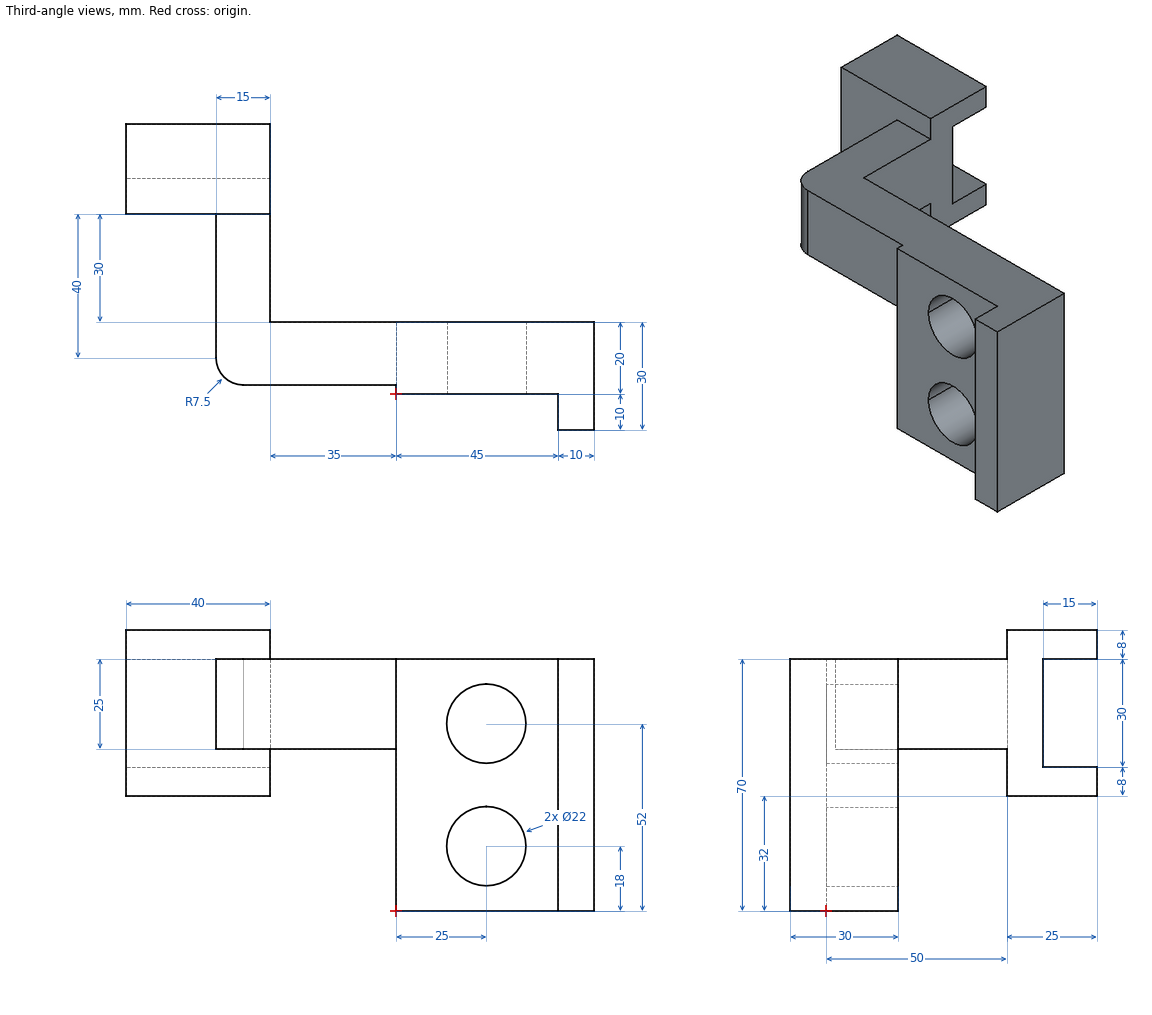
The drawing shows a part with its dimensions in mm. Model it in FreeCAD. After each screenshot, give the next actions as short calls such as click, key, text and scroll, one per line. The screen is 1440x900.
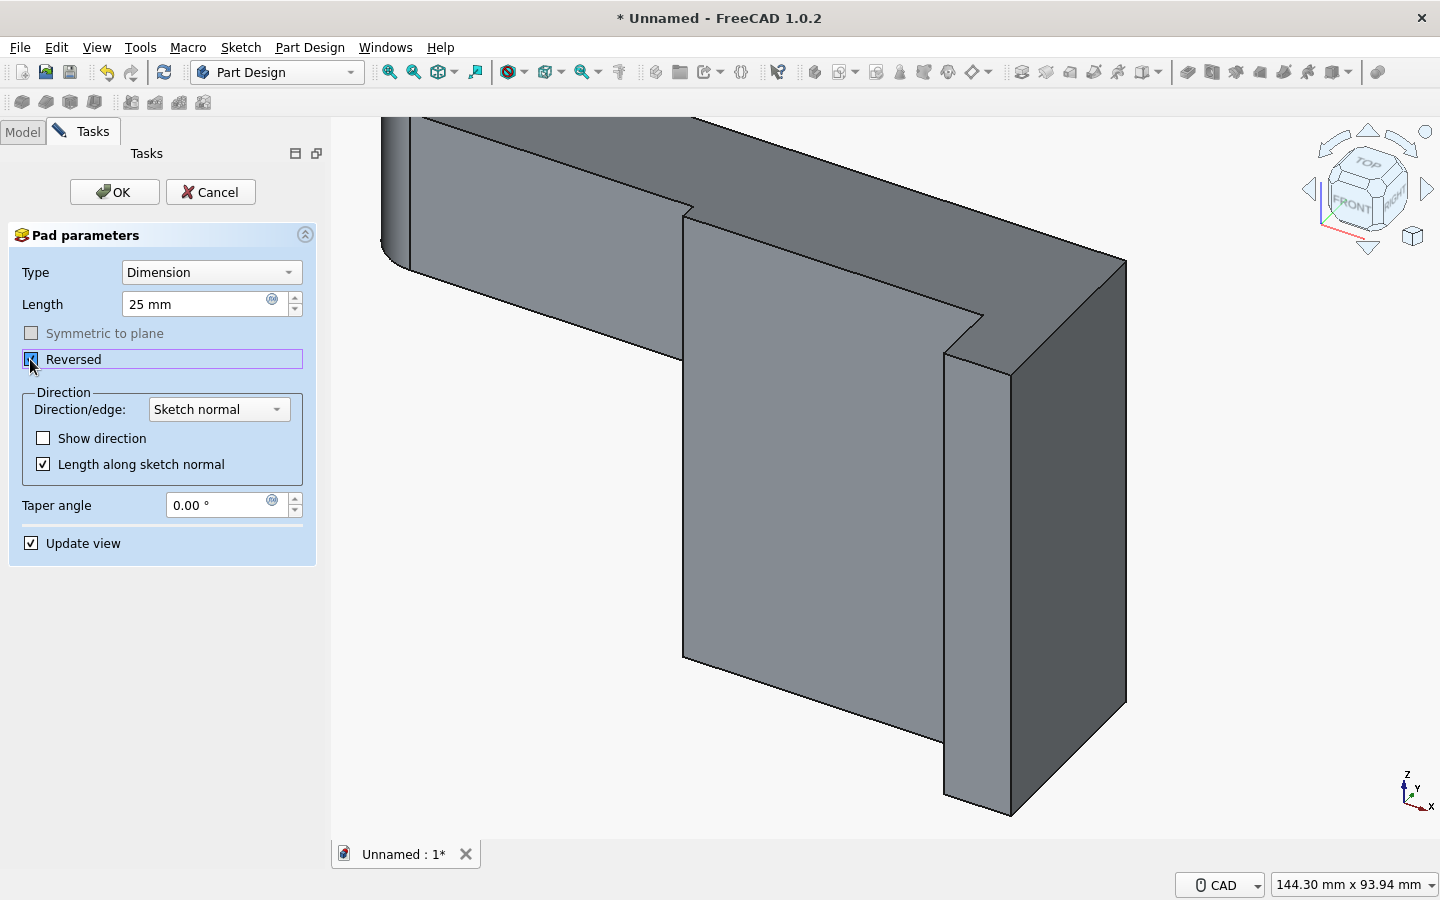
click(115, 192)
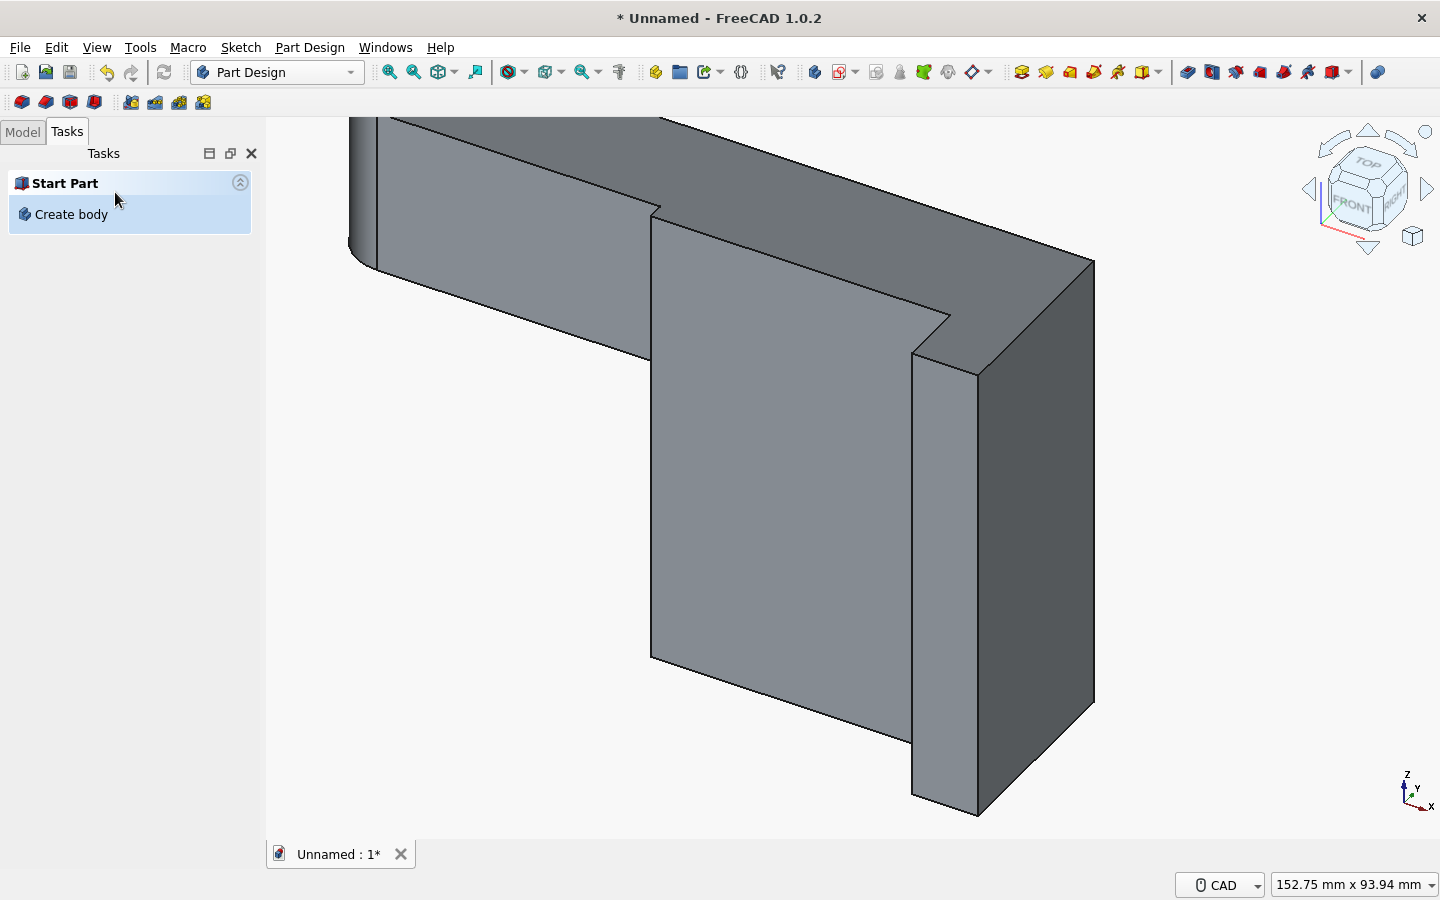
click(390, 72)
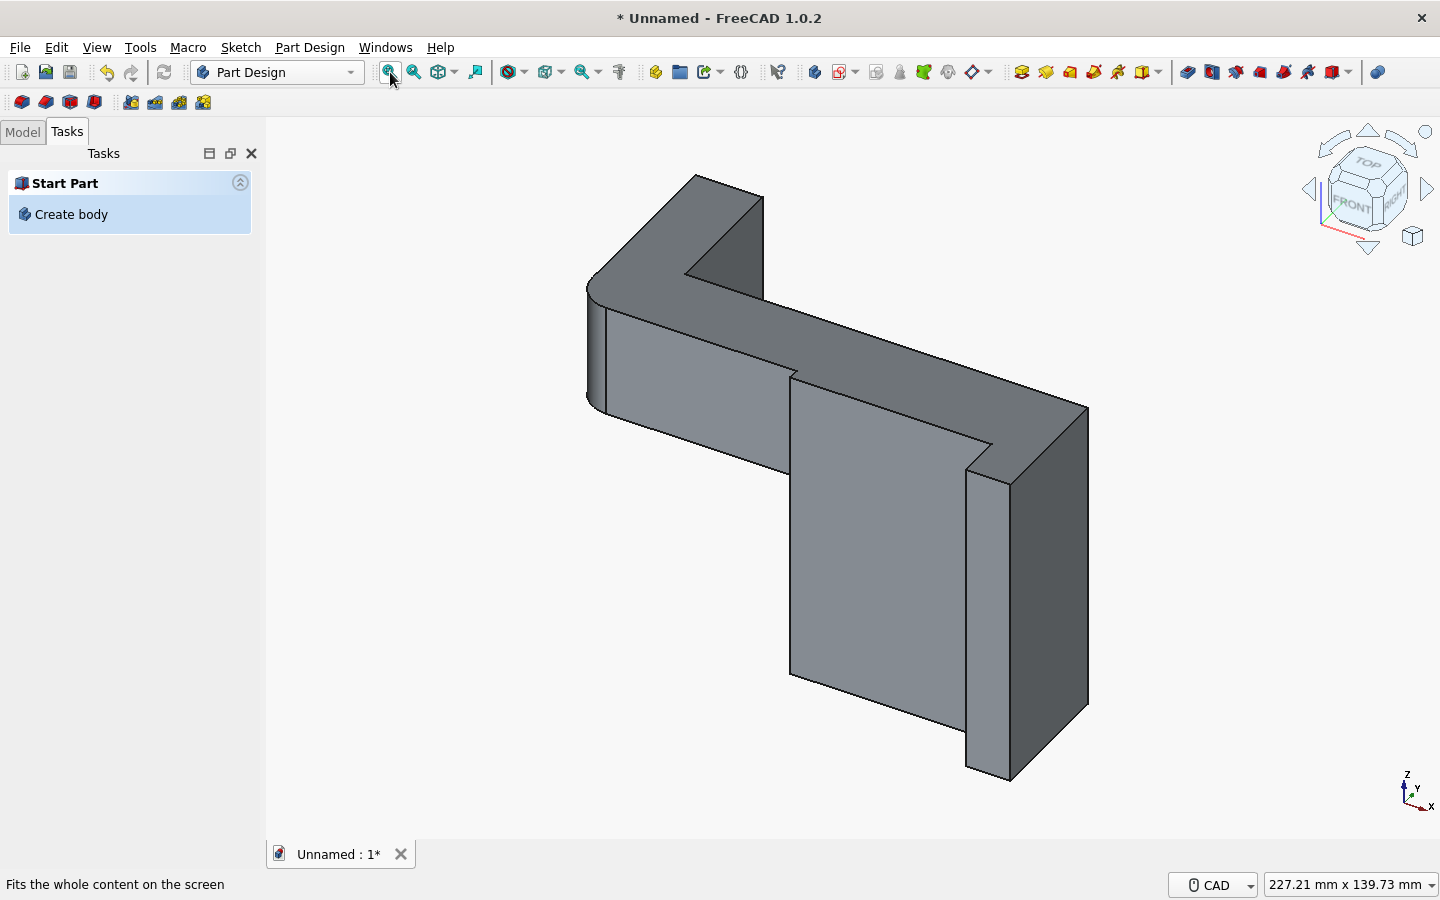
click(735, 277)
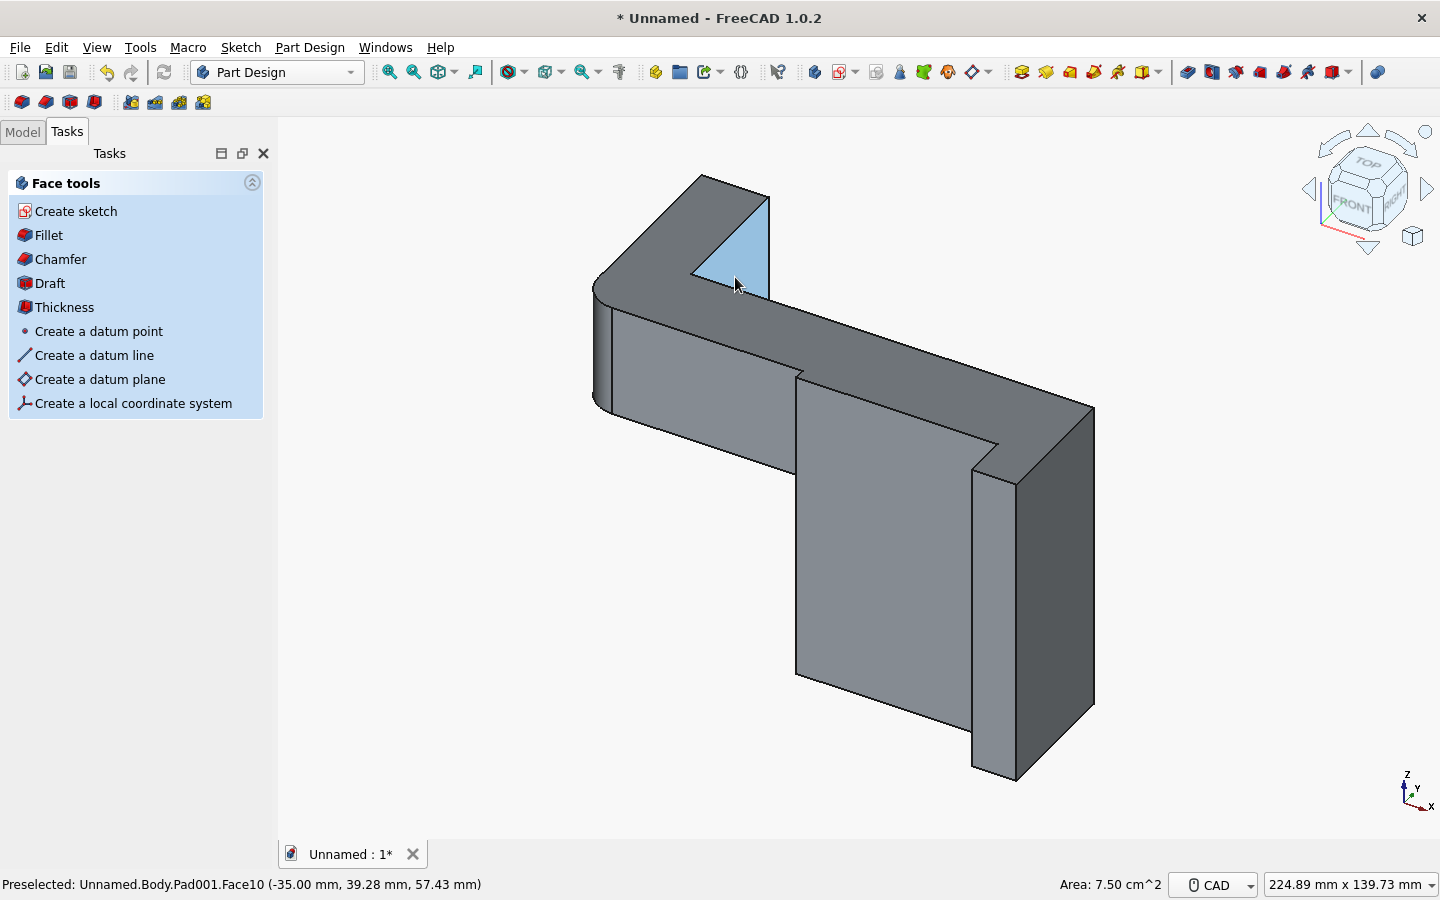
click(840, 72)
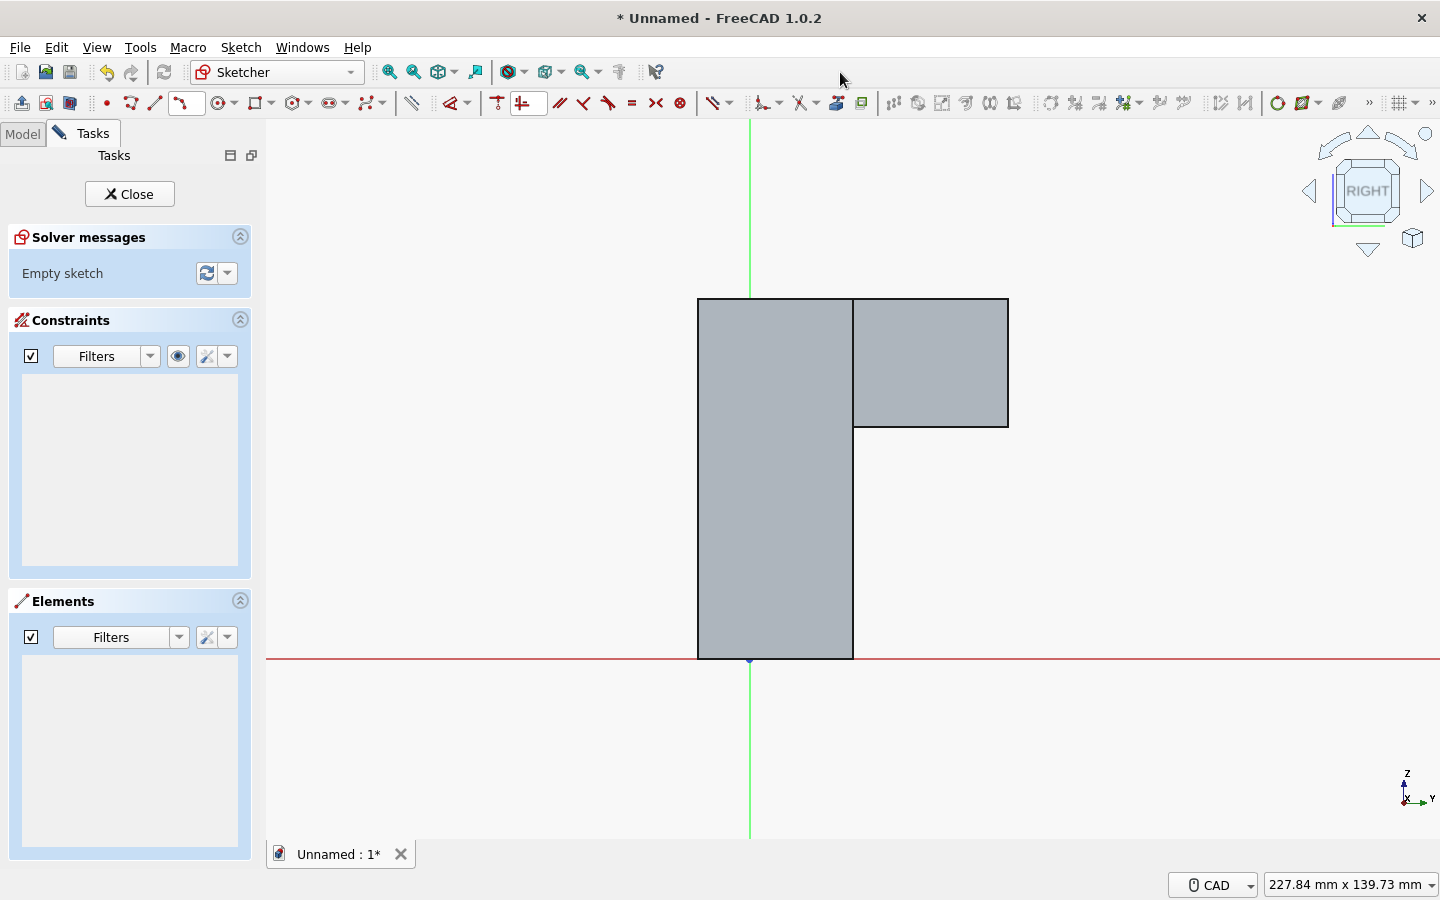
click(132, 104)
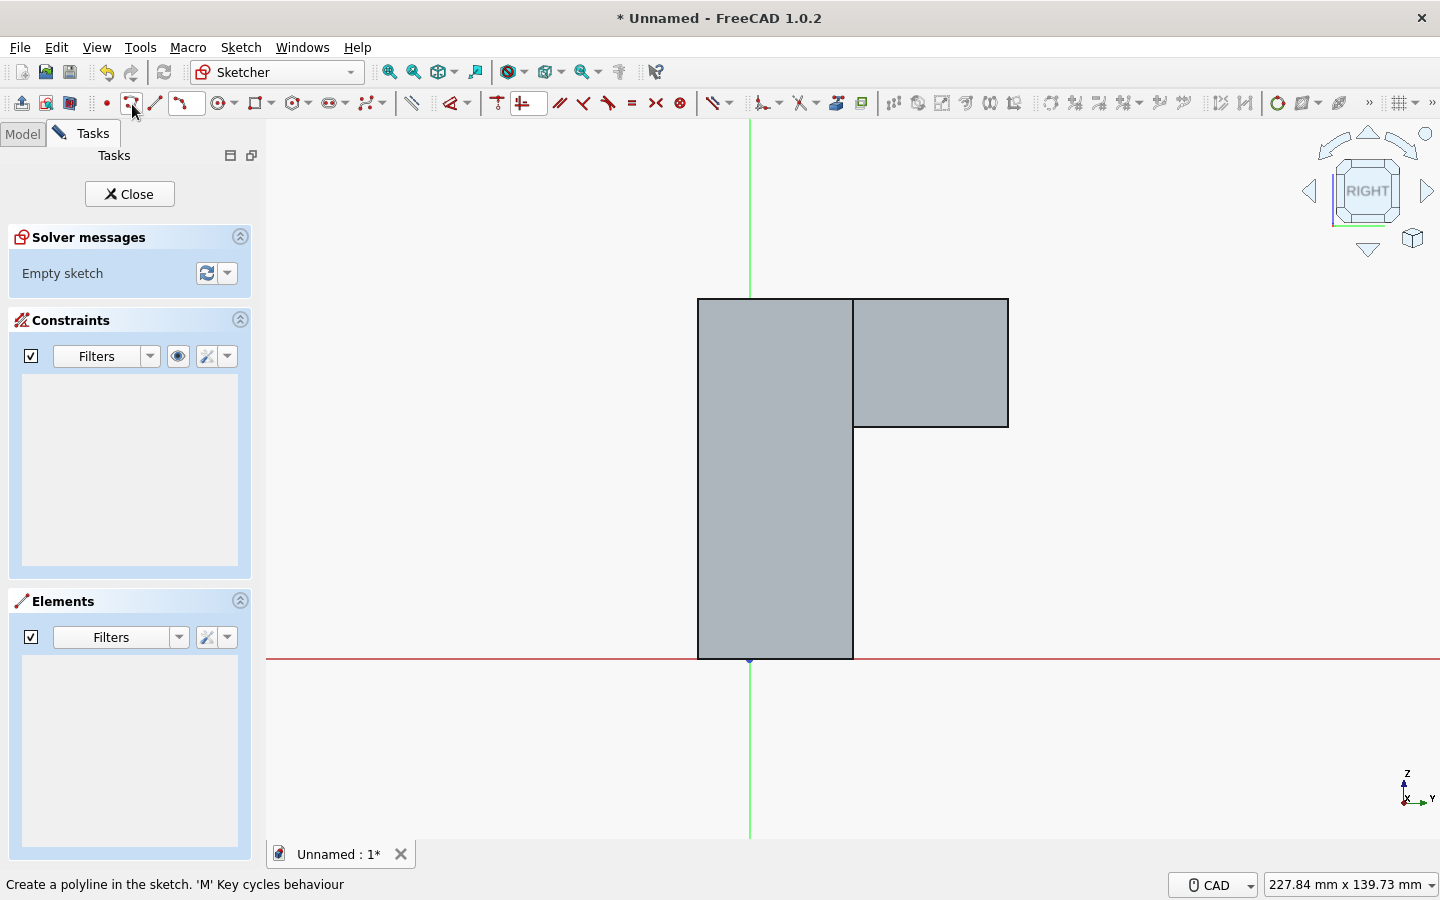
click(1008, 494)
click(1136, 494)
click(1136, 453)
click(1059, 453)
click(1059, 299)
click(1136, 299)
click(1136, 257)
click(1008, 257)
click(1008, 495)
key(Escape)
key(Escape)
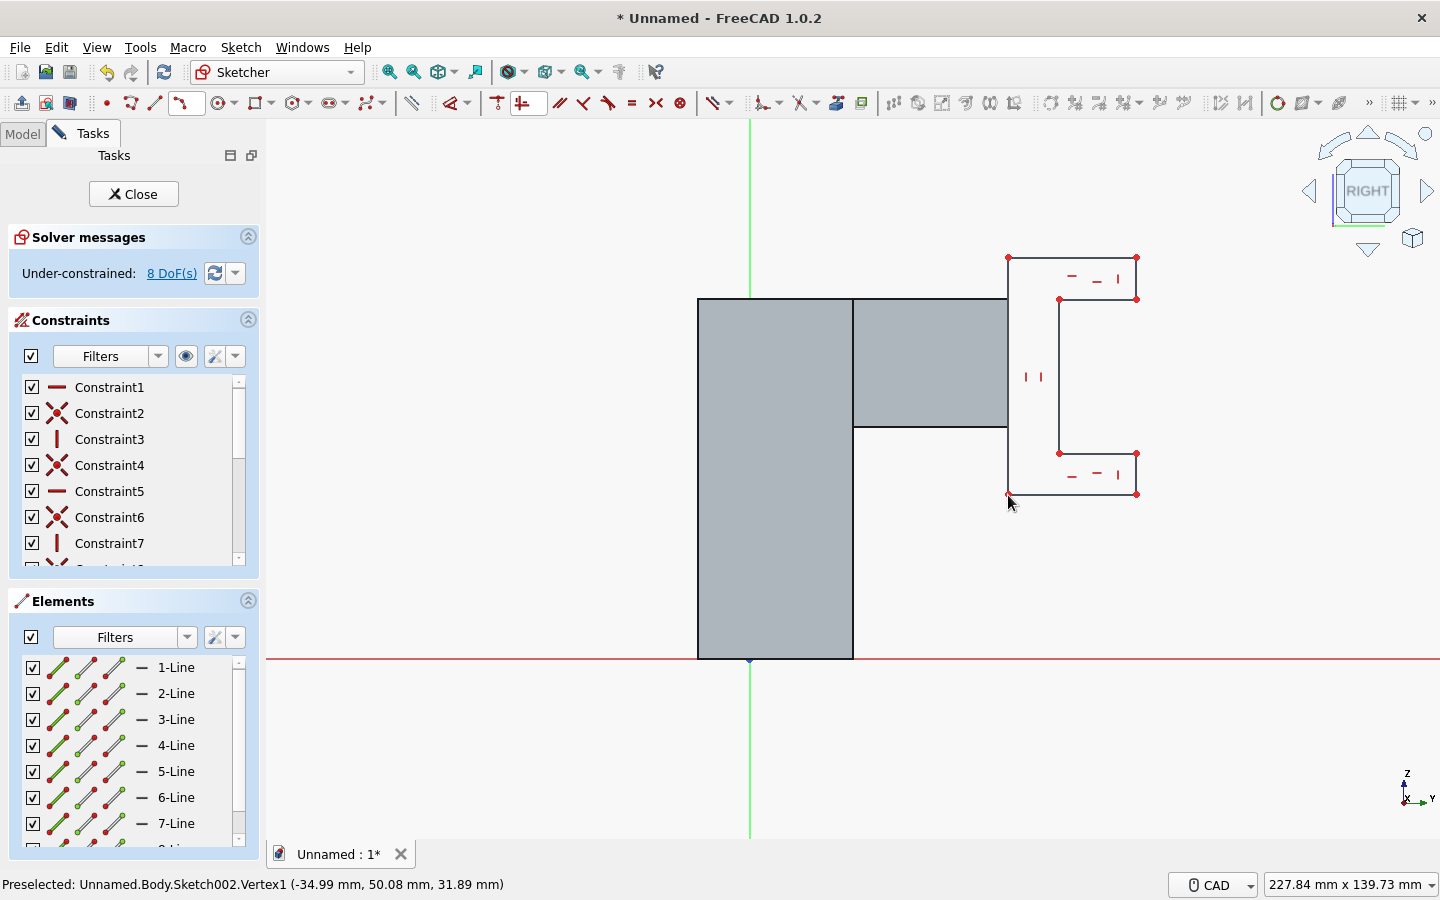
click(450, 104)